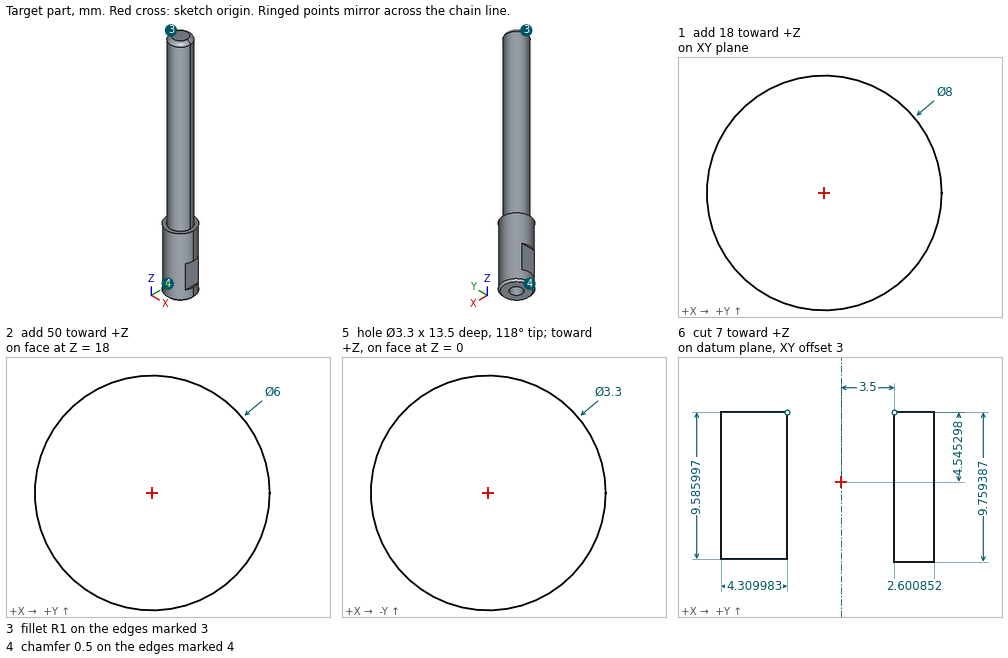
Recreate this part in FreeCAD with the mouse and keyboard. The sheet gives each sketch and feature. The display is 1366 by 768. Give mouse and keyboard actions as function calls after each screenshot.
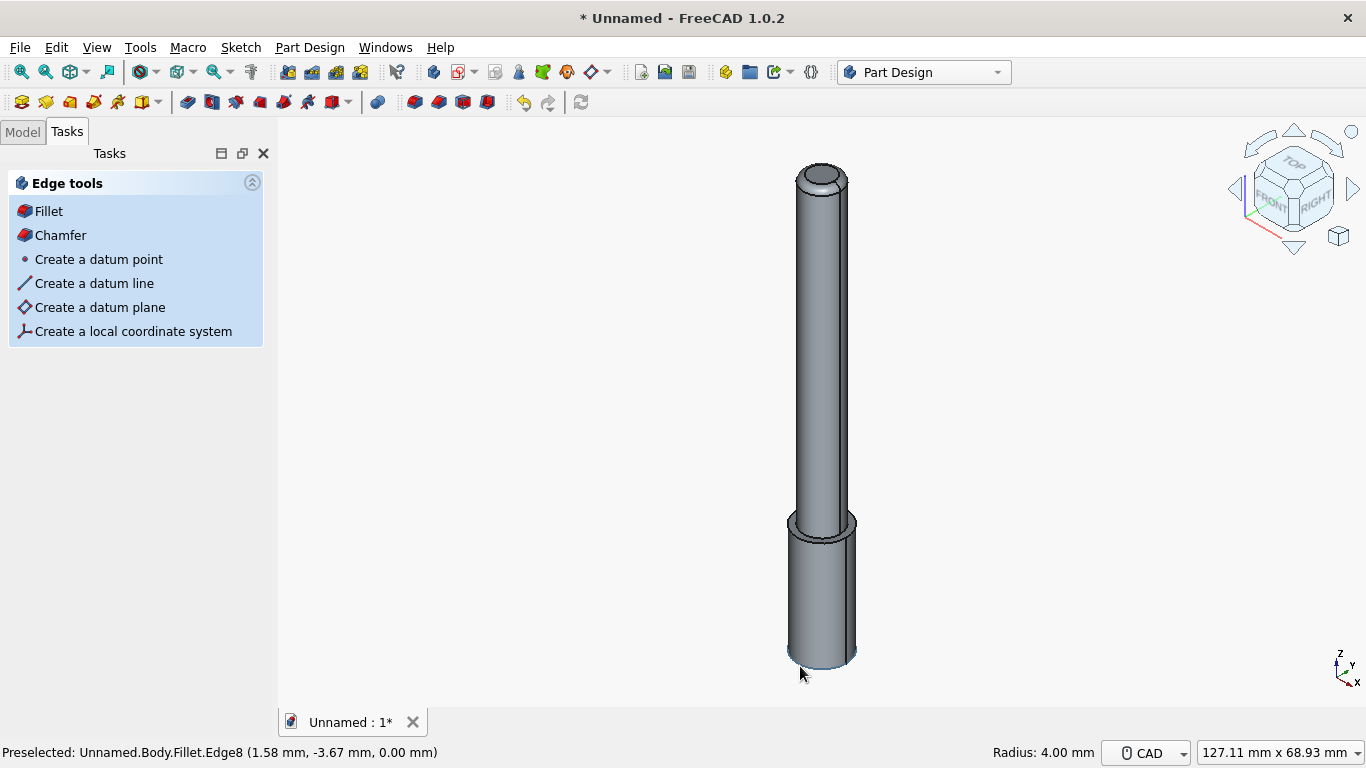
click(440, 102)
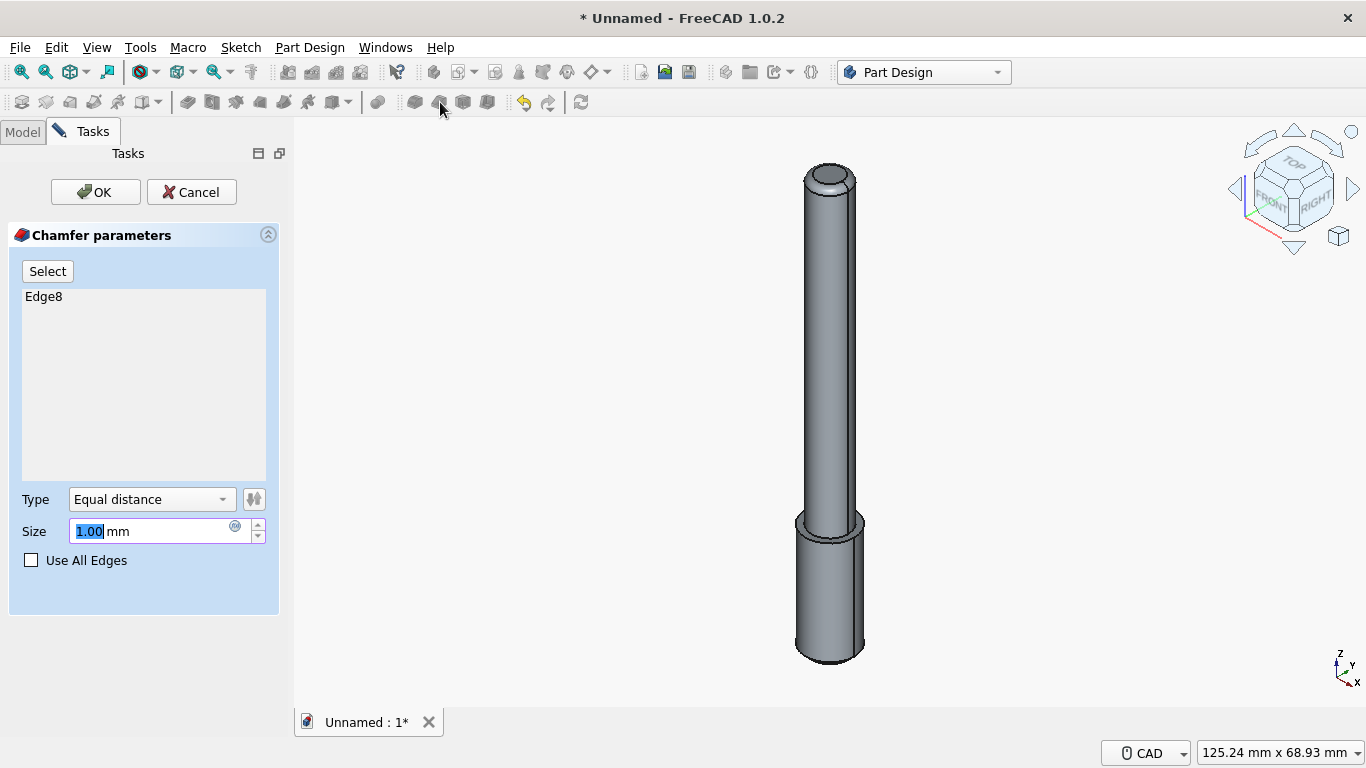
text(0.5)
key(Tab)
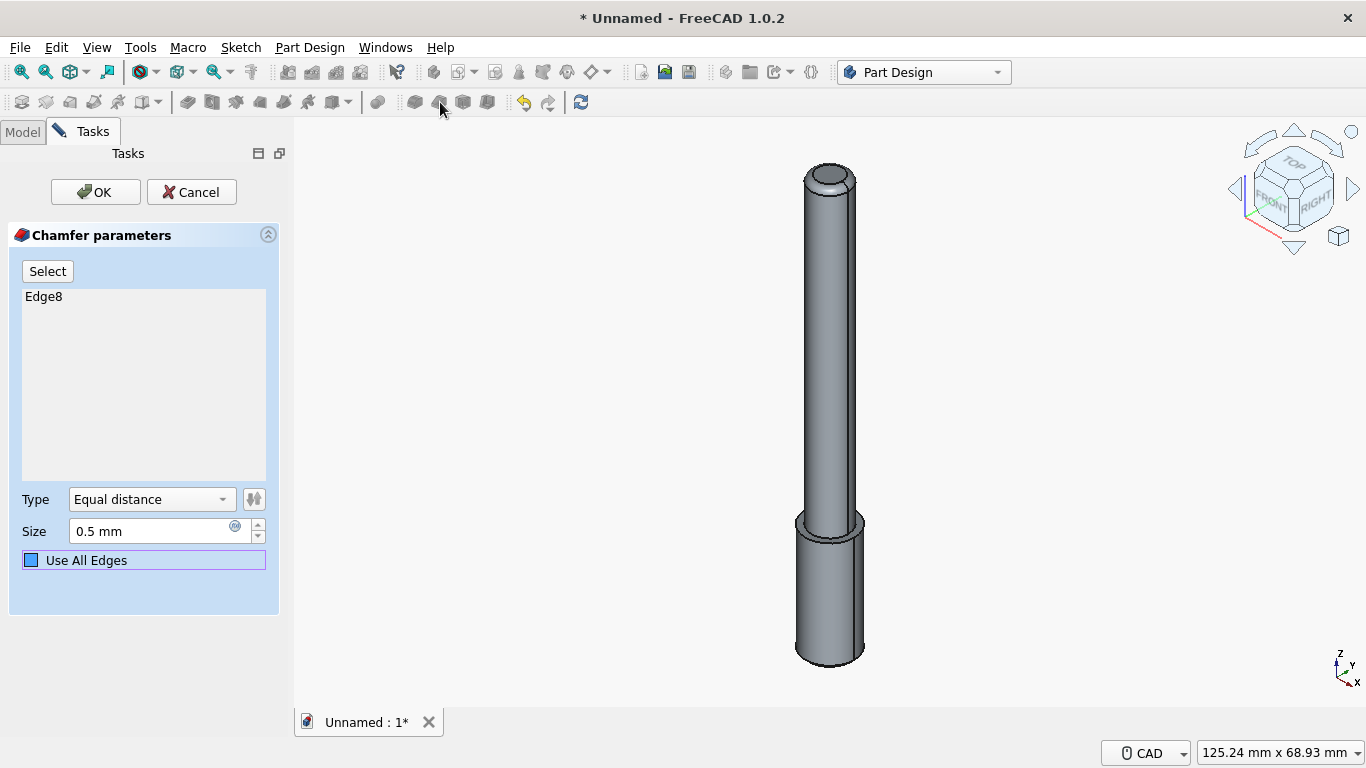
click(96, 192)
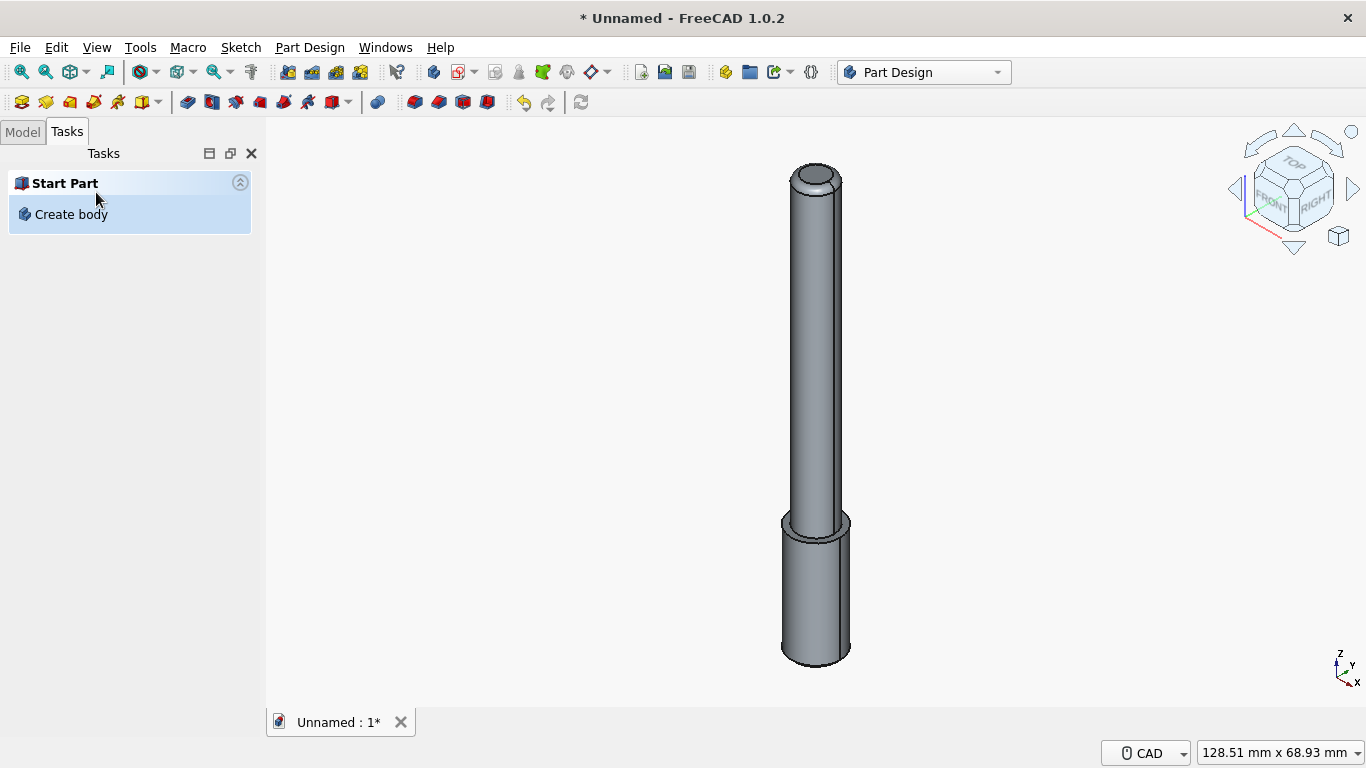
key(5)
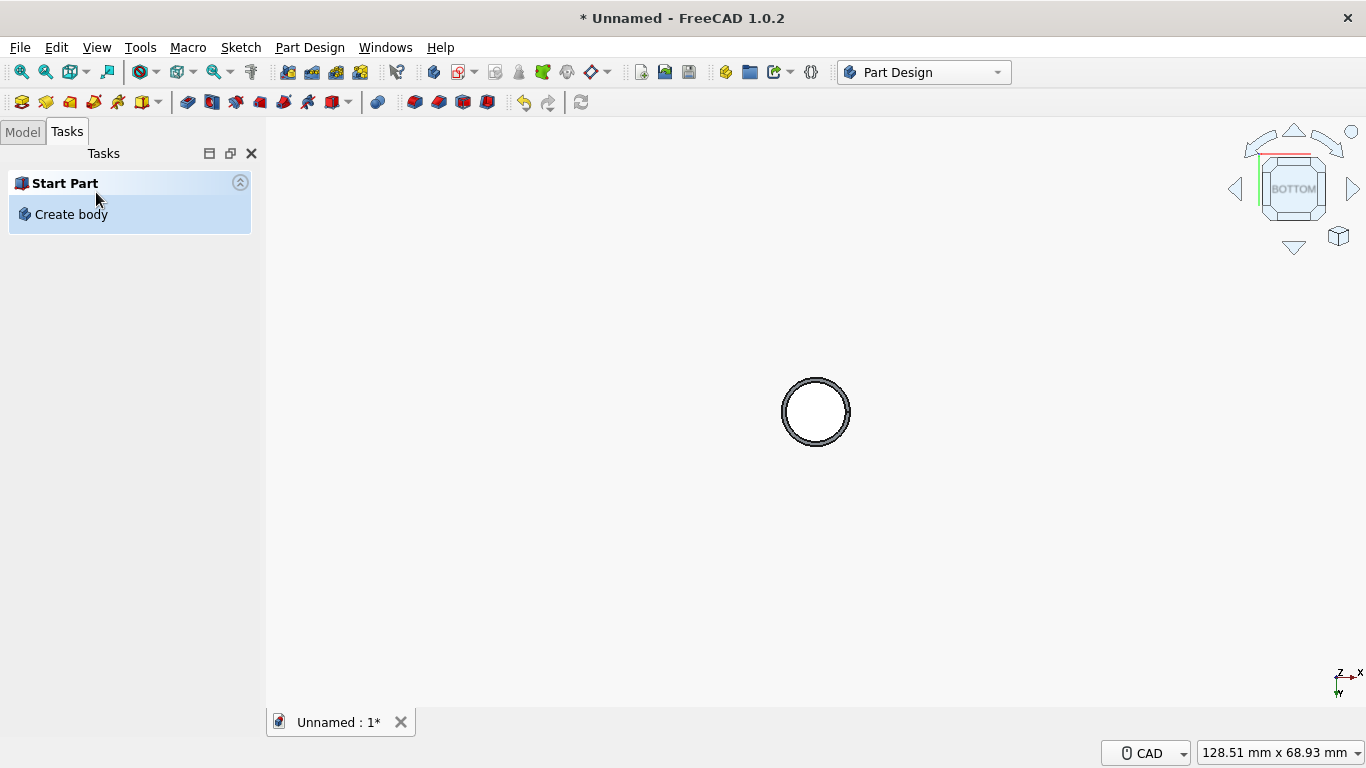
click(22, 72)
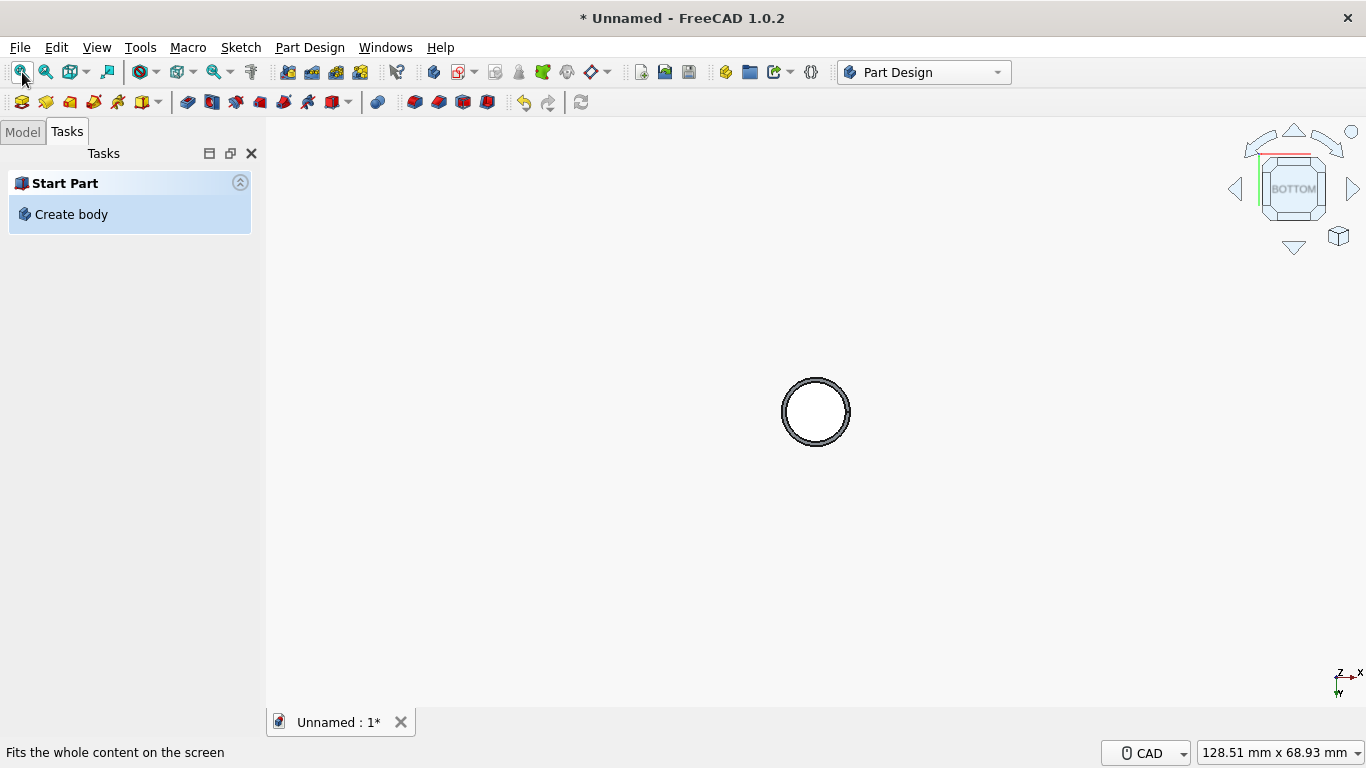
click(816, 411)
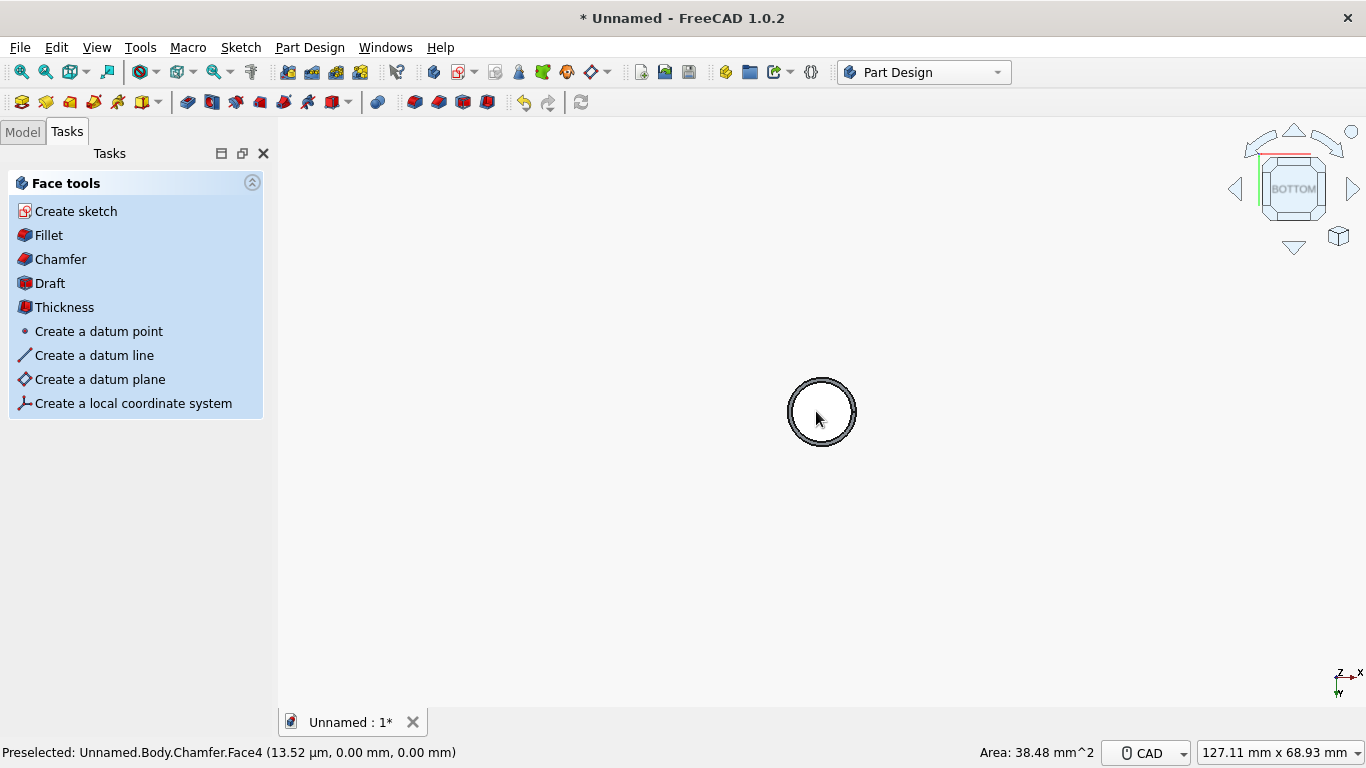
click(458, 72)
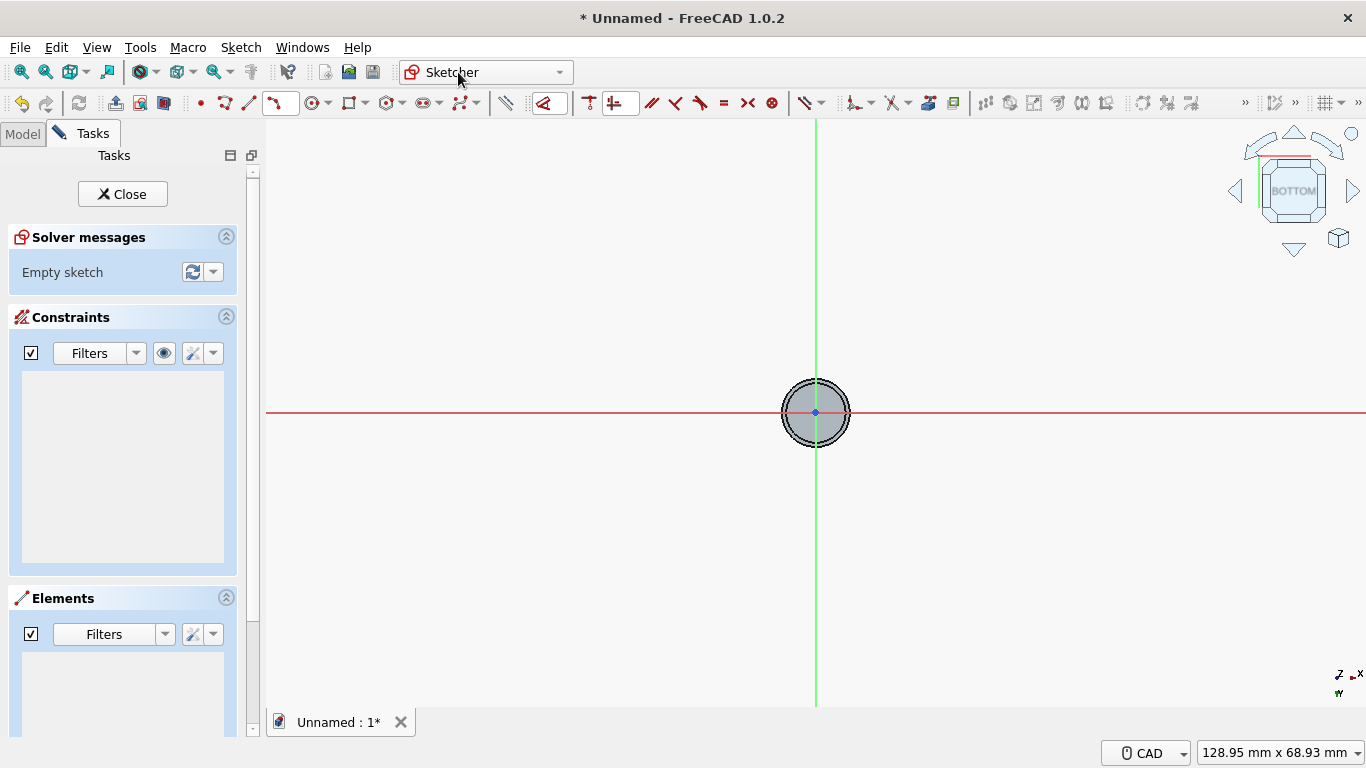
scroll(821, 413, up, 13)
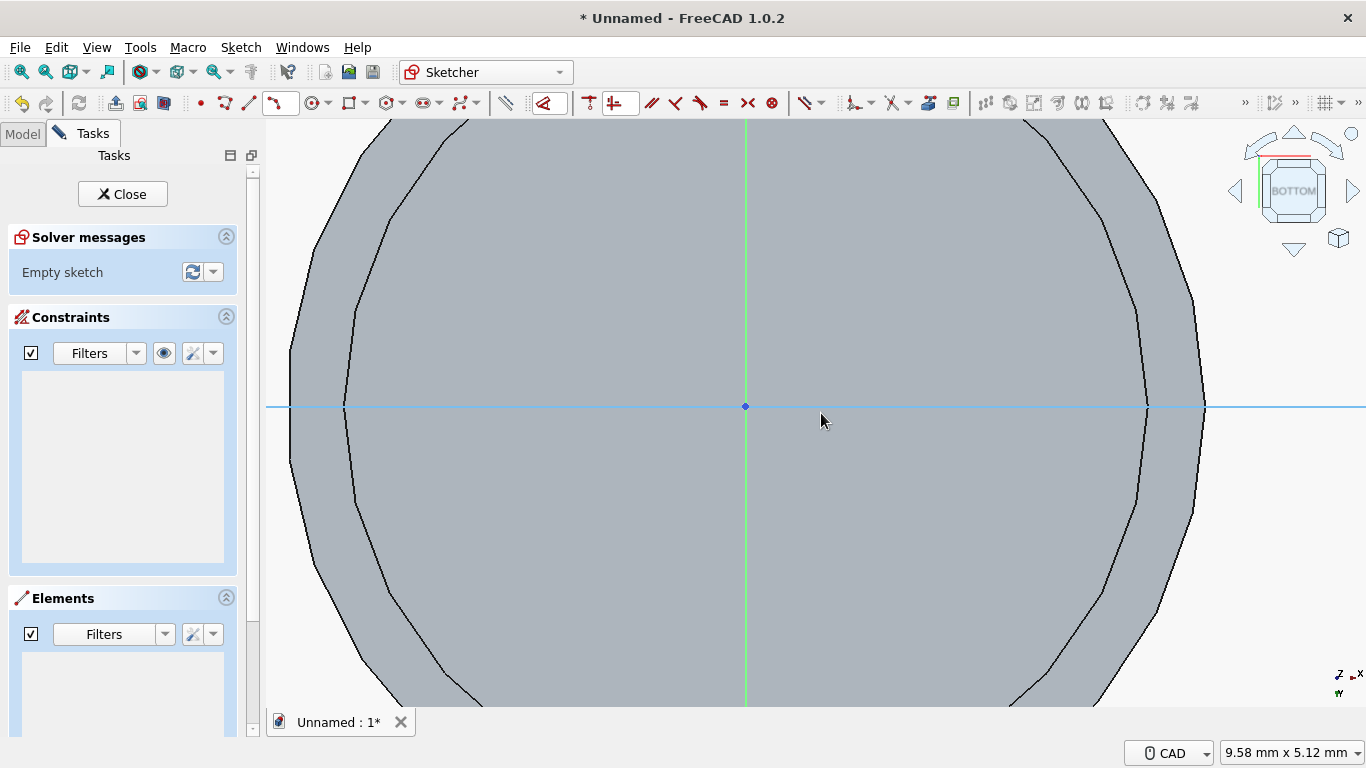
click(312, 104)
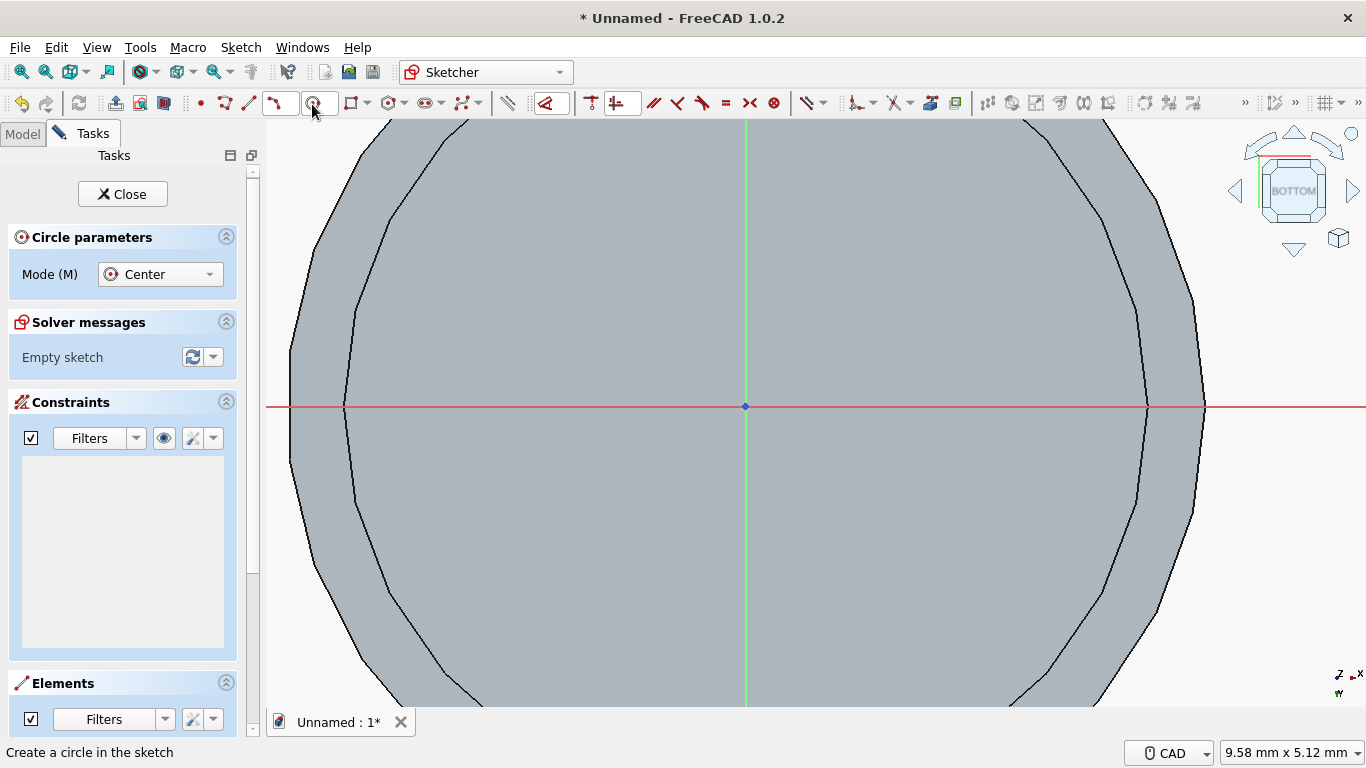
click(746, 407)
move(880, 273)